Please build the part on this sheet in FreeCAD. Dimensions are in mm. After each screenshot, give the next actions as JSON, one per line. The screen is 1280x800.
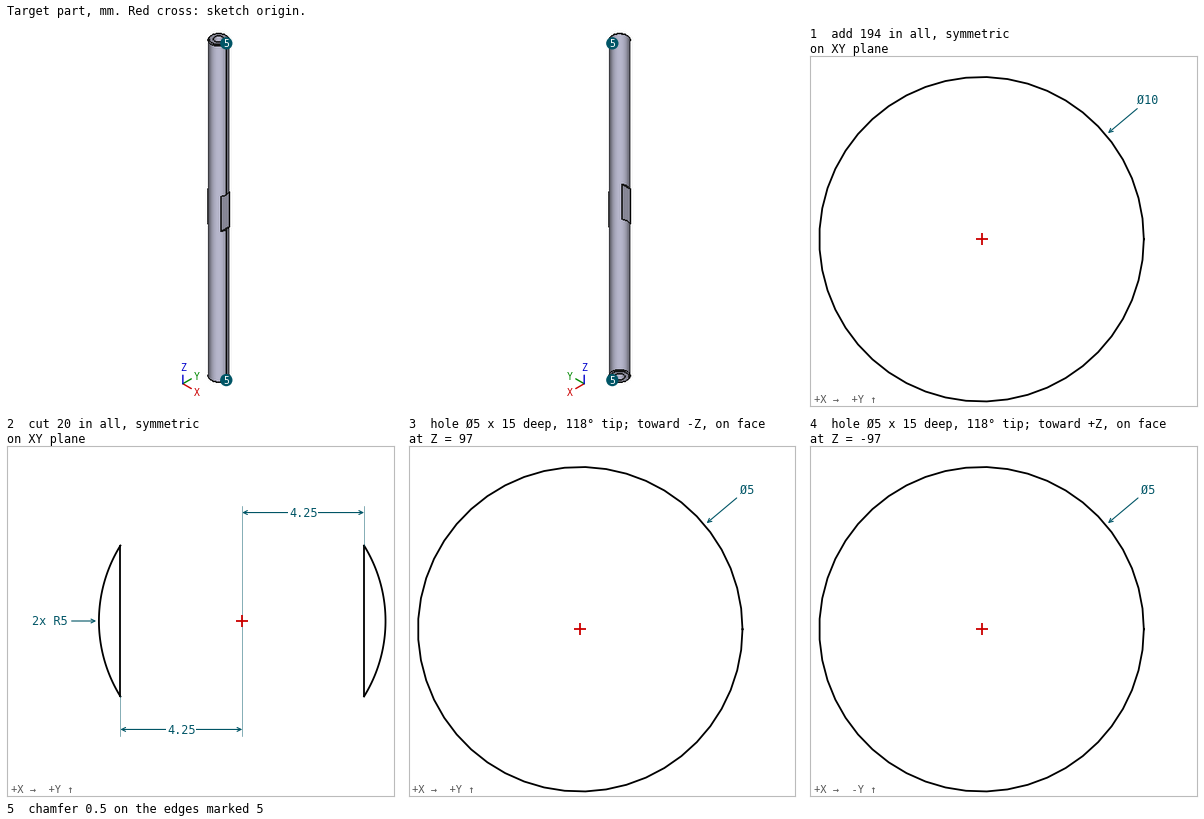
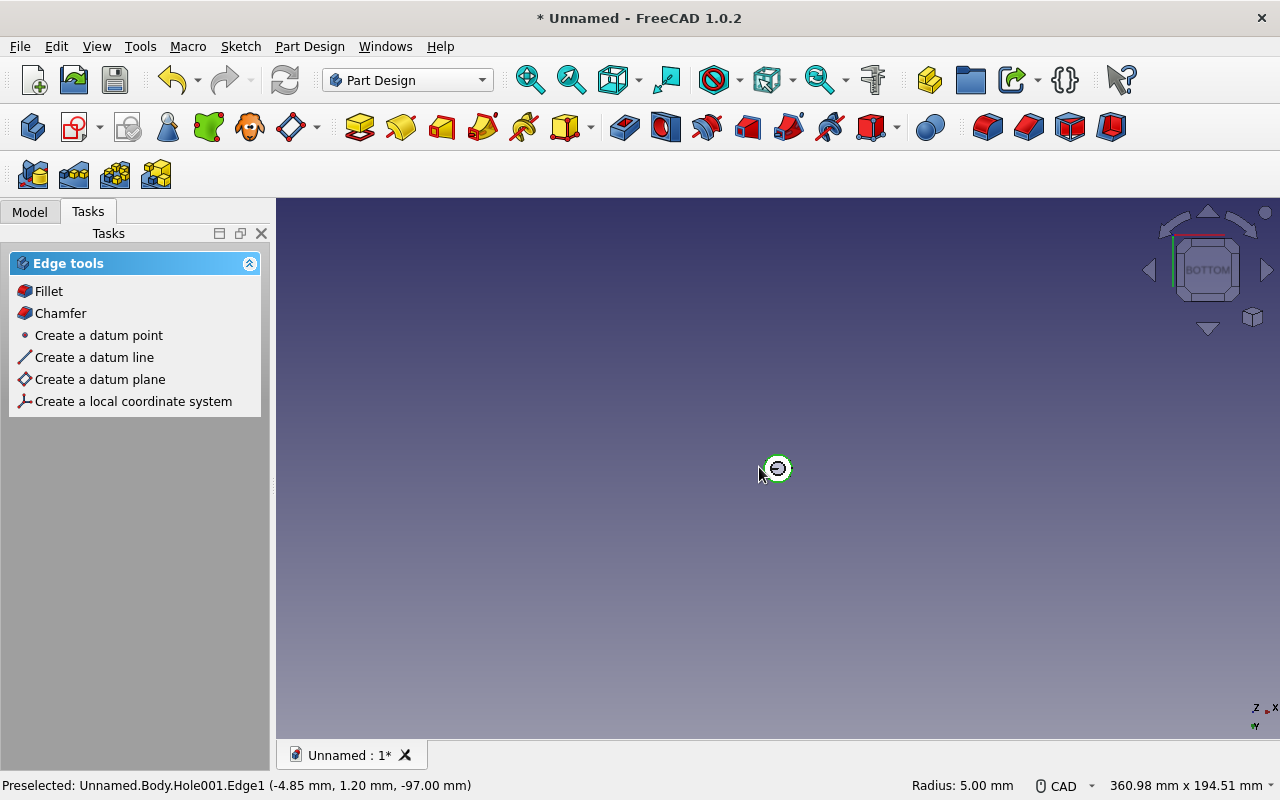
{"action": "key", "text": "0"}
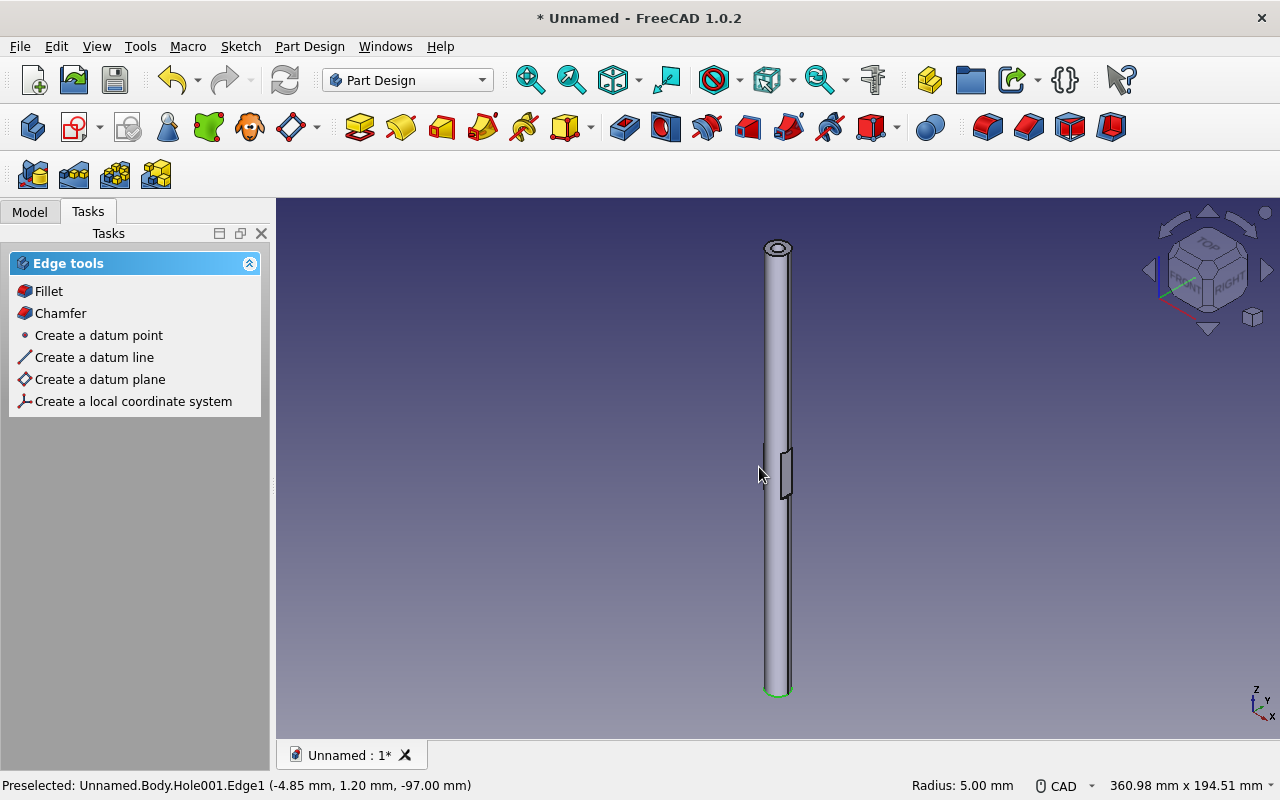
{"action": "left_click", "coordinate": [764, 246], "text": "ctrl"}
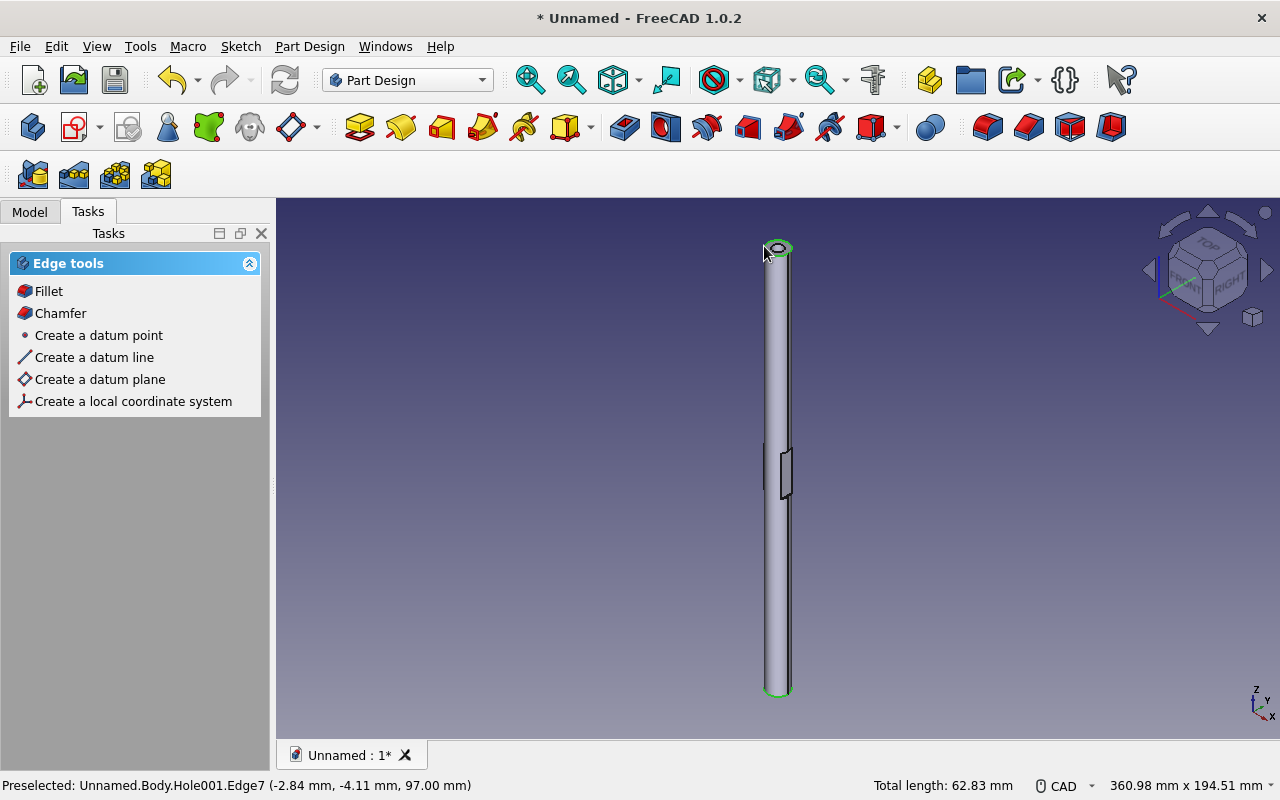
{"action": "left_click", "coordinate": [1029, 128]}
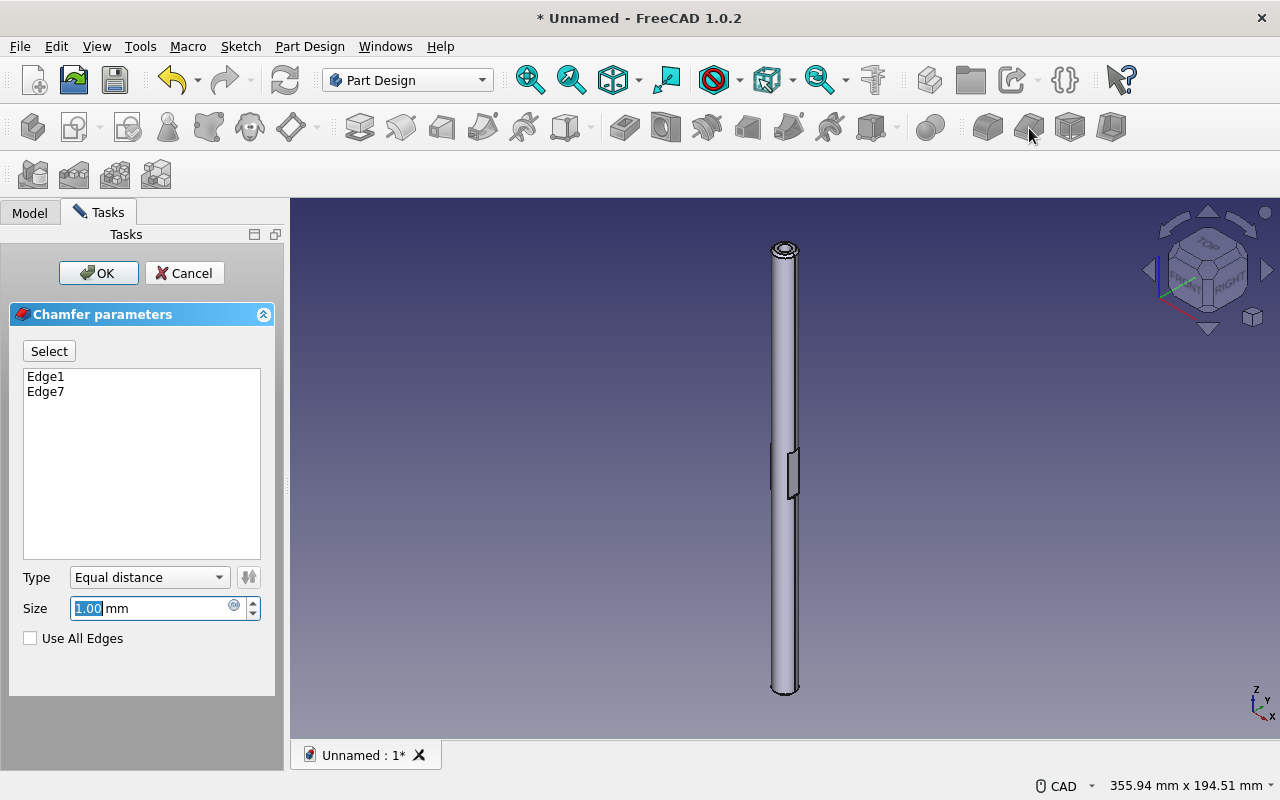
{"action": "type", "text": "0.5"}
{"action": "key", "text": "Tab"}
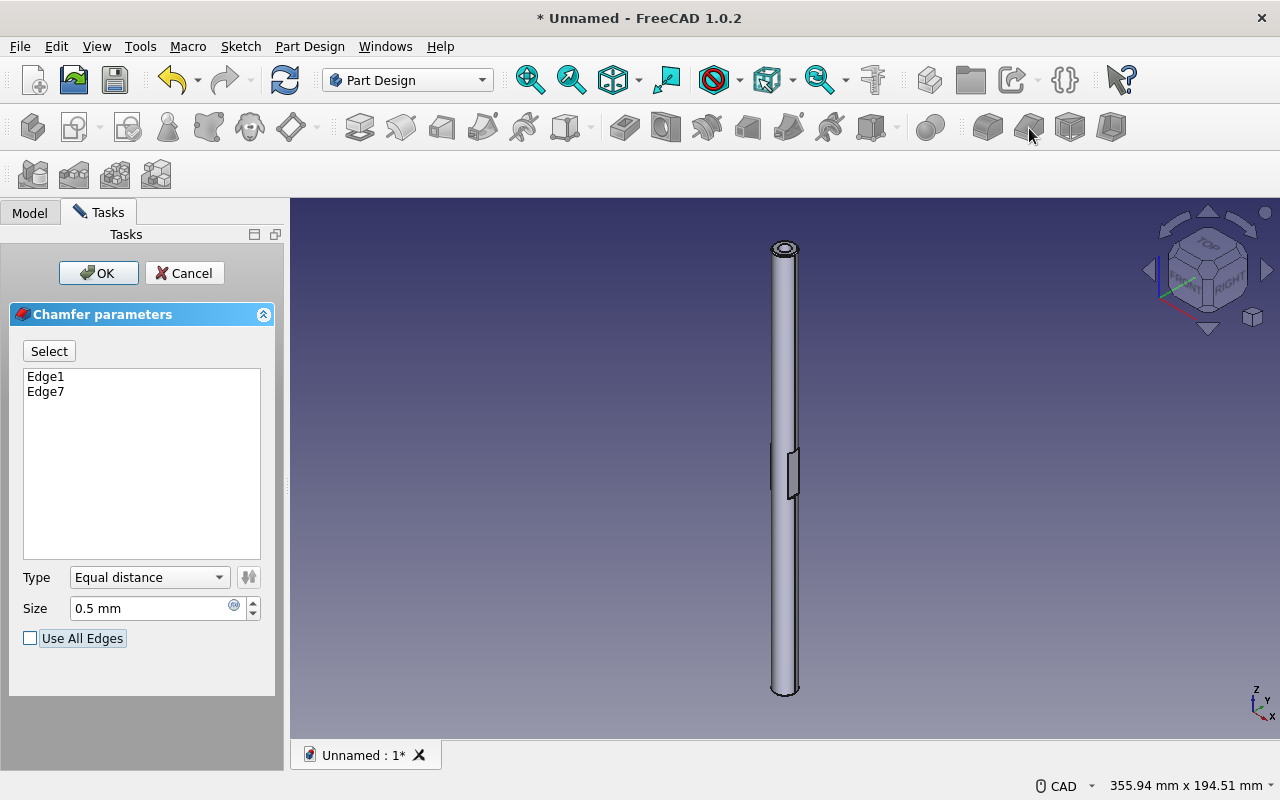
{"action": "left_click", "coordinate": [99, 273]}